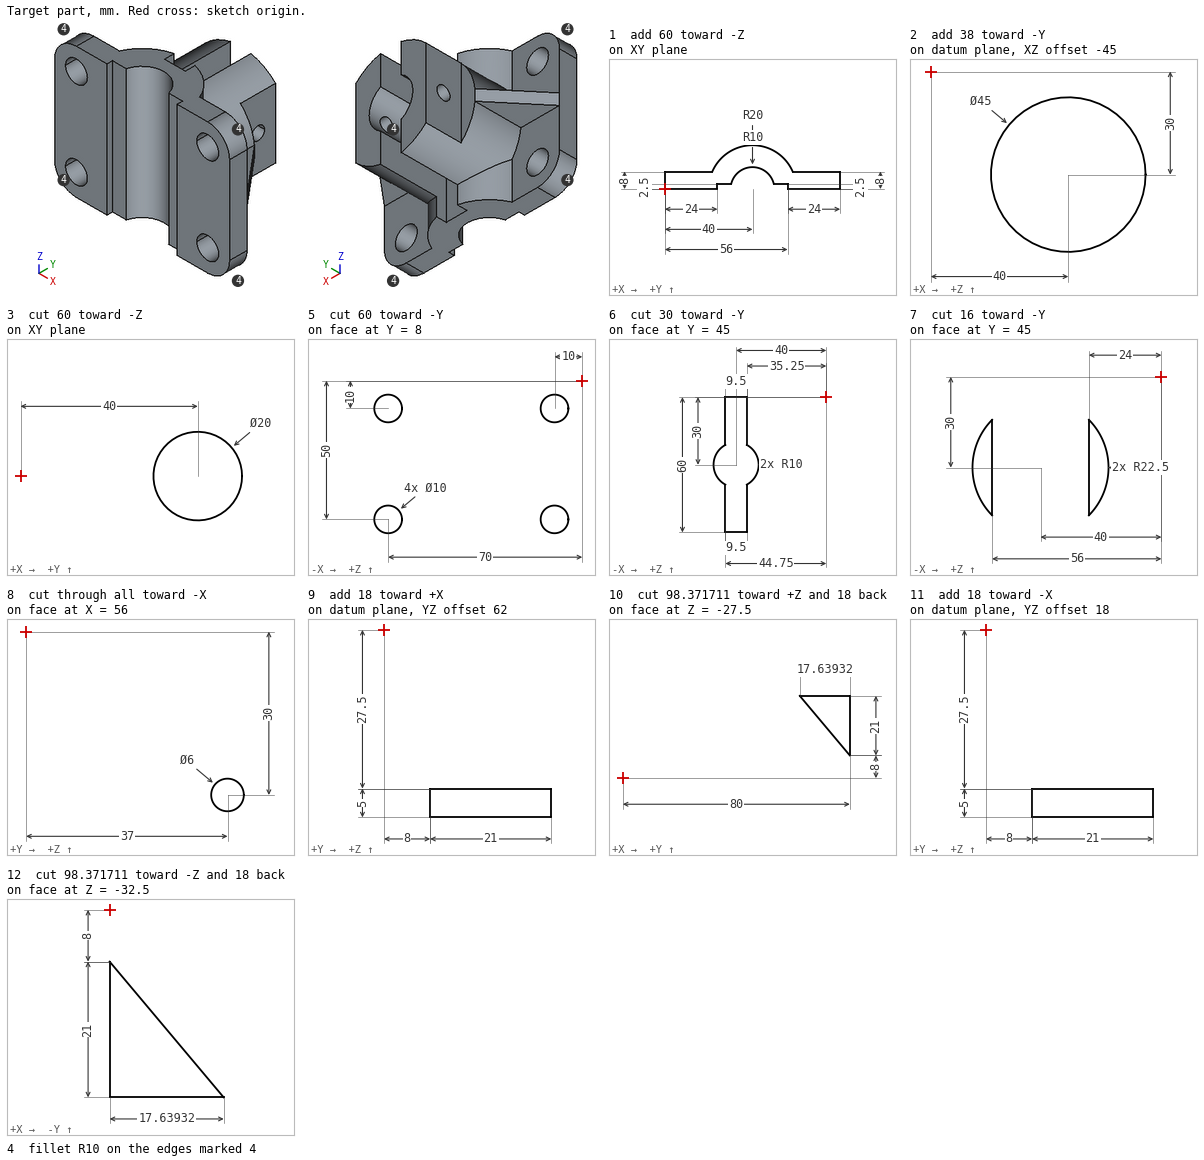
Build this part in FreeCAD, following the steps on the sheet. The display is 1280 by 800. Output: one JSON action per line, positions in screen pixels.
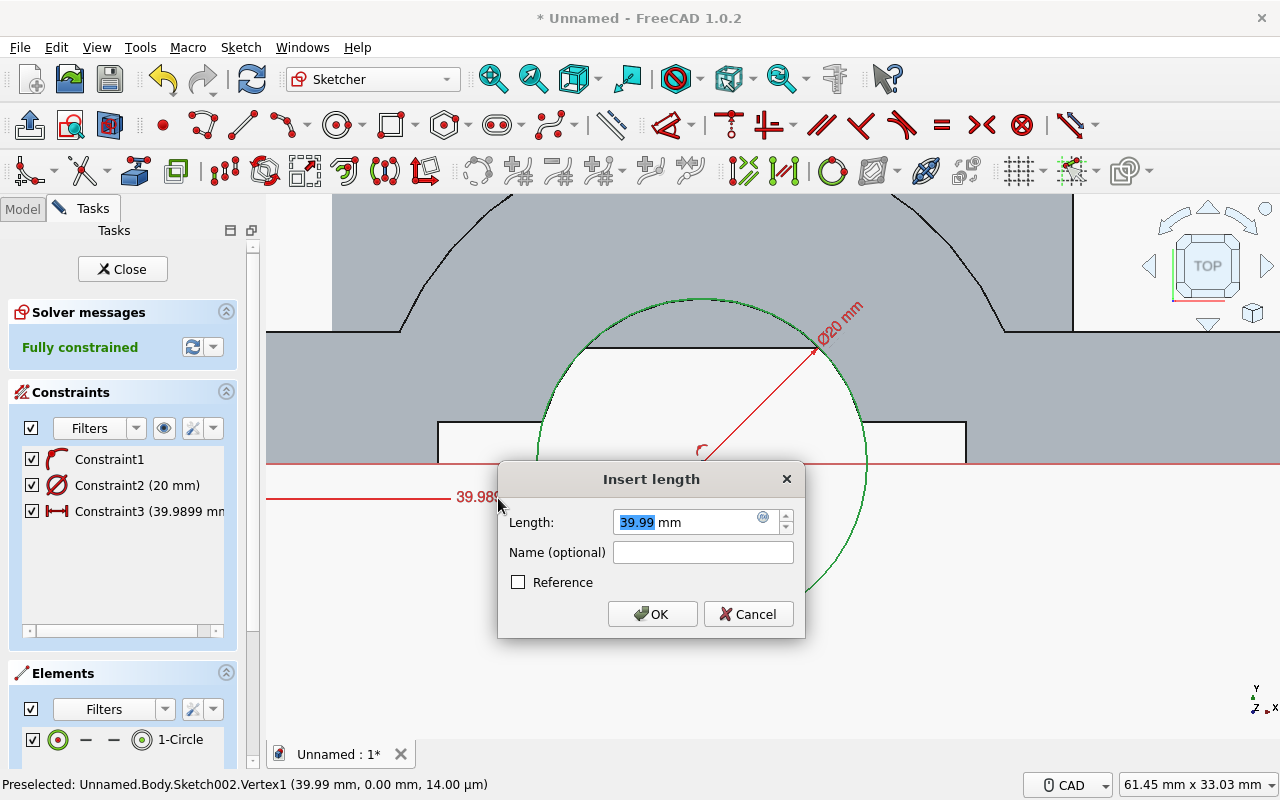
{"action": "type", "text": "40"}
{"action": "key", "text": "Return"}
{"action": "key", "text": "Escape"}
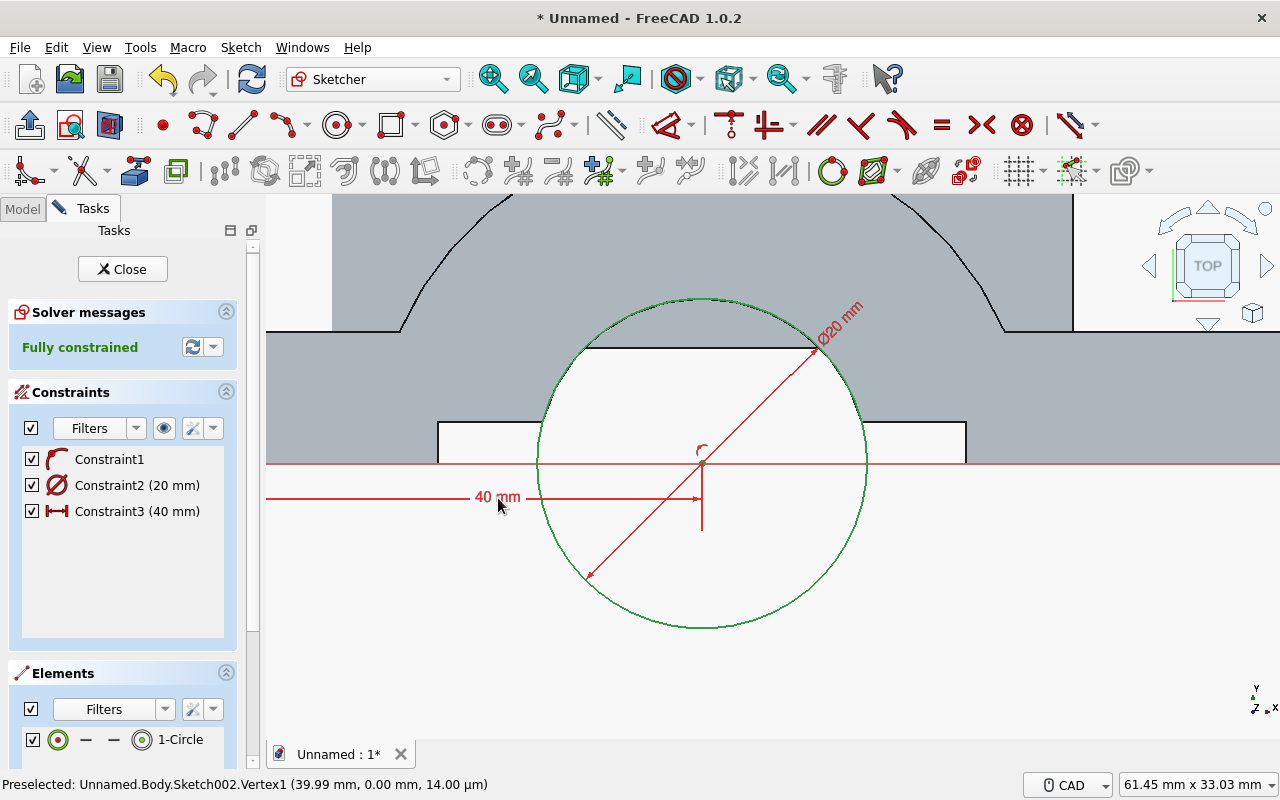
{"action": "left_click", "coordinate": [123, 269]}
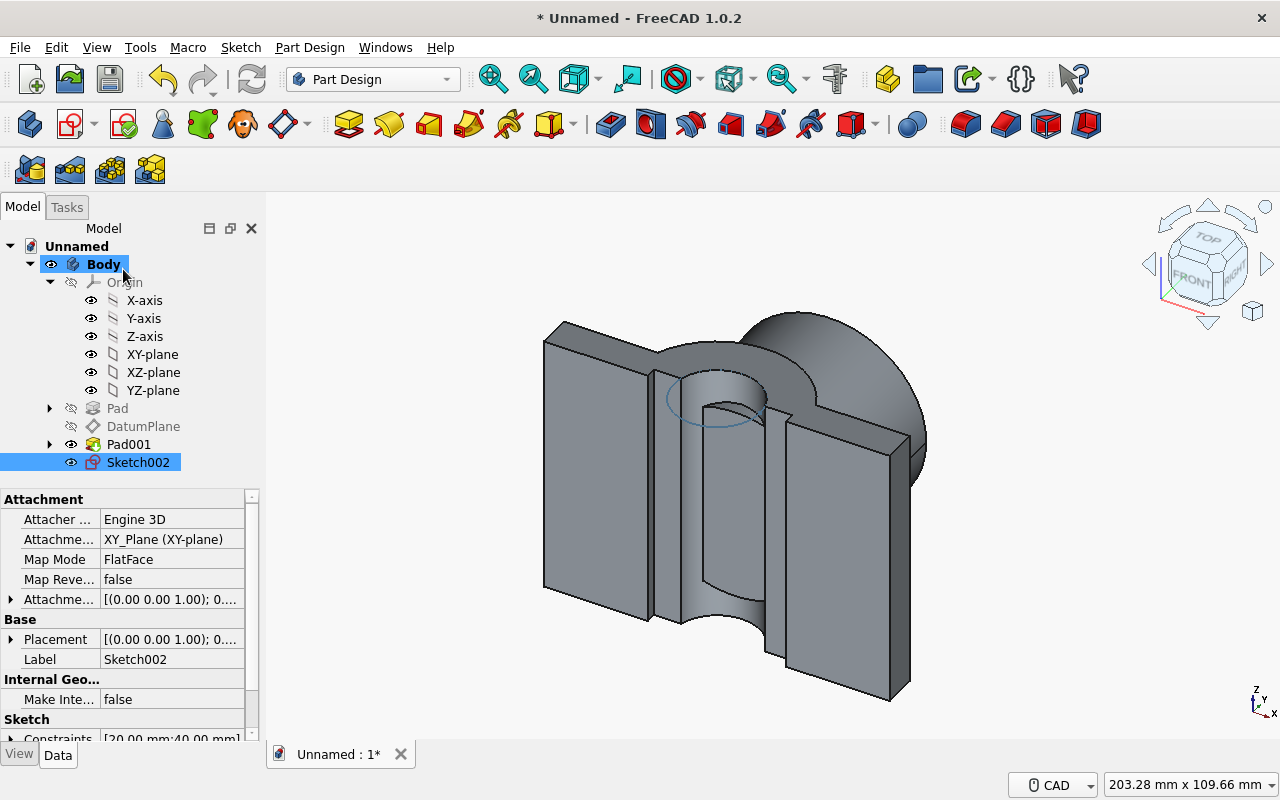
{"action": "left_click", "coordinate": [612, 124]}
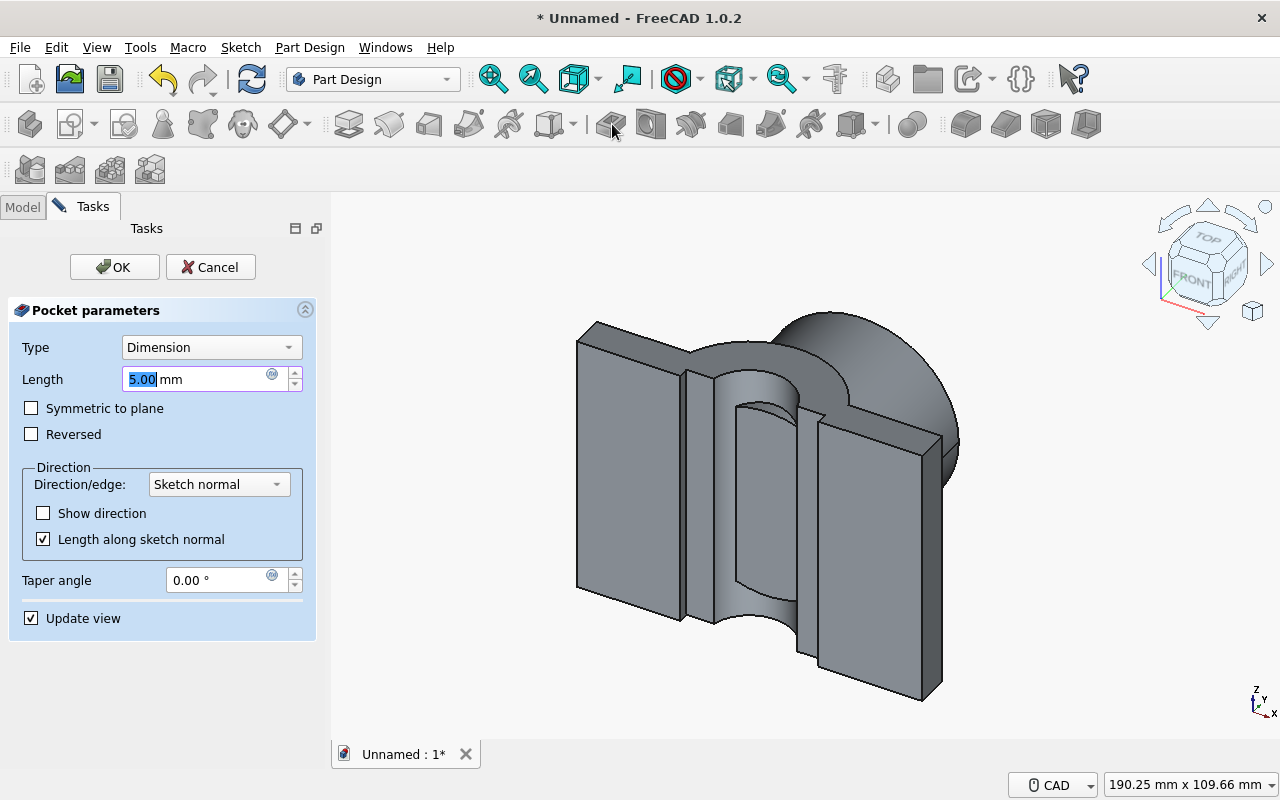
{"action": "type", "text": "60"}
{"action": "key", "text": "Tab"}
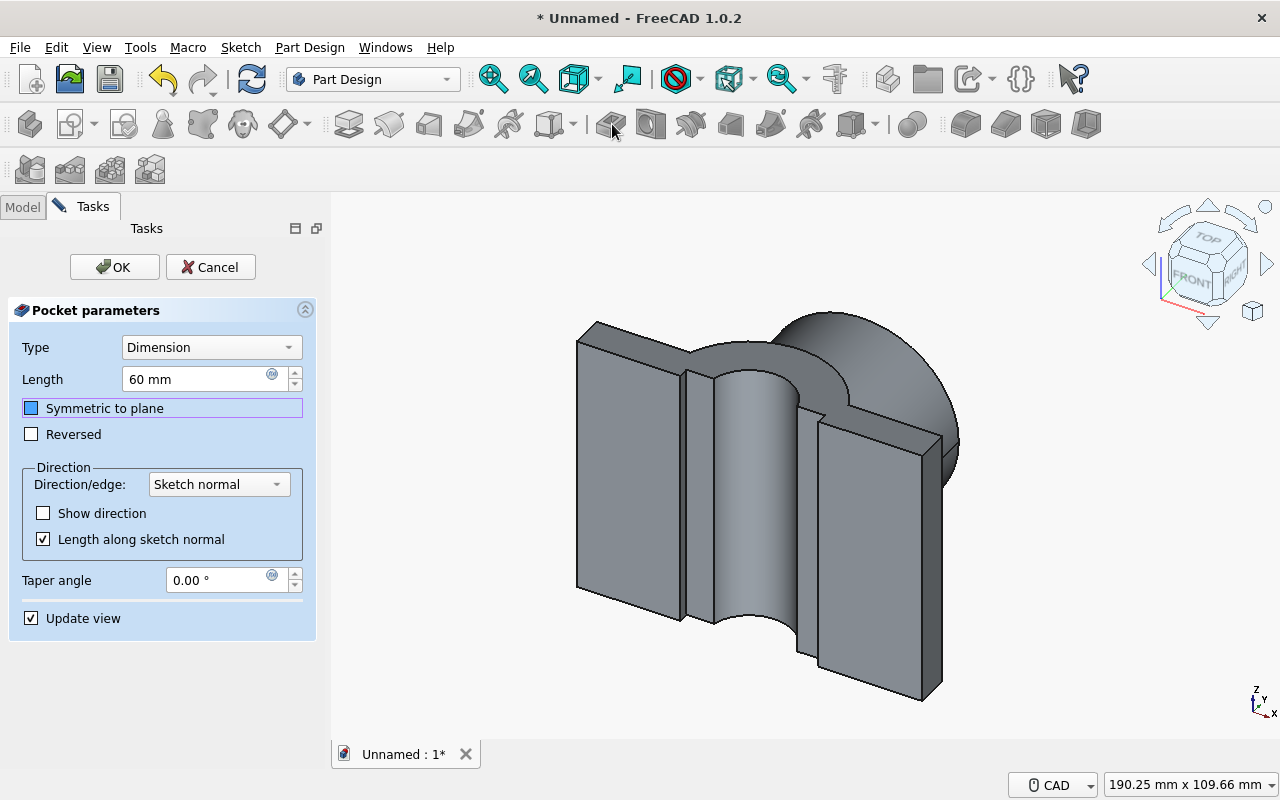
{"action": "left_click", "coordinate": [115, 267]}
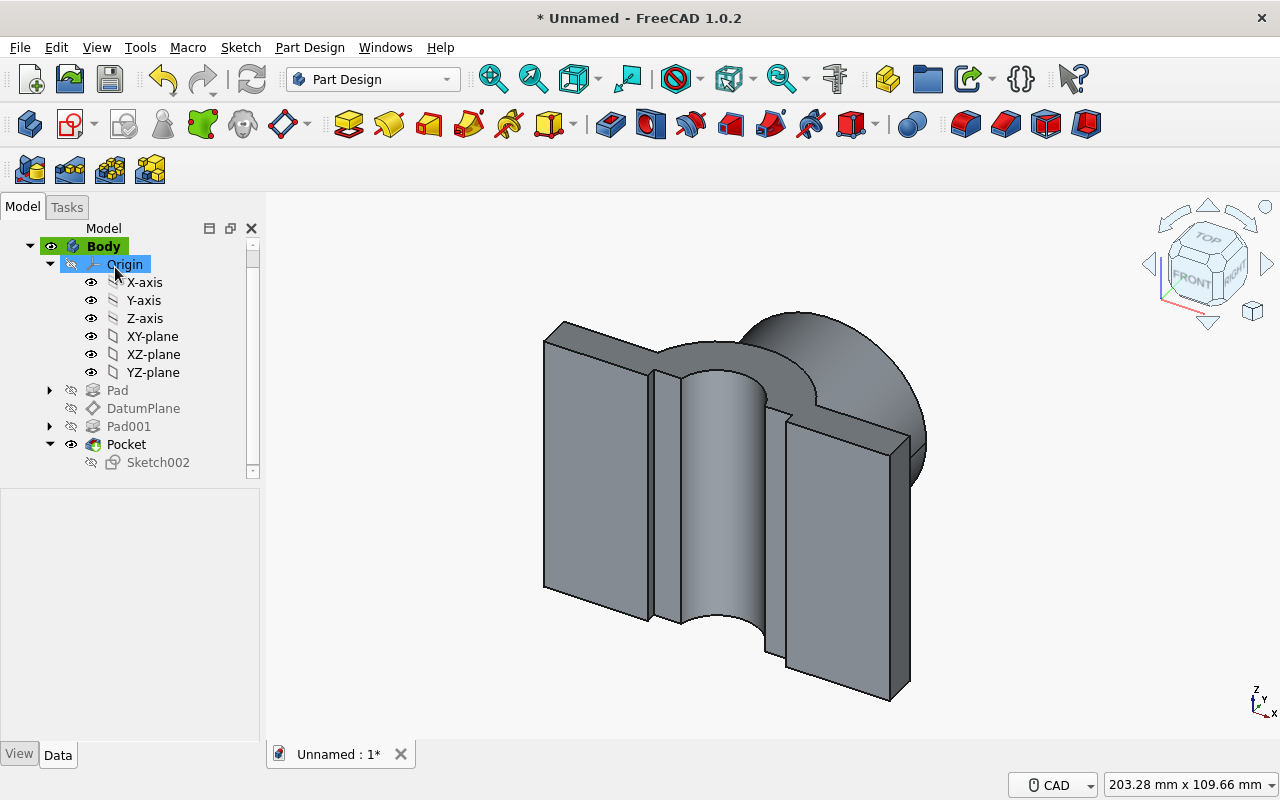
{"action": "left_click", "coordinate": [900, 445]}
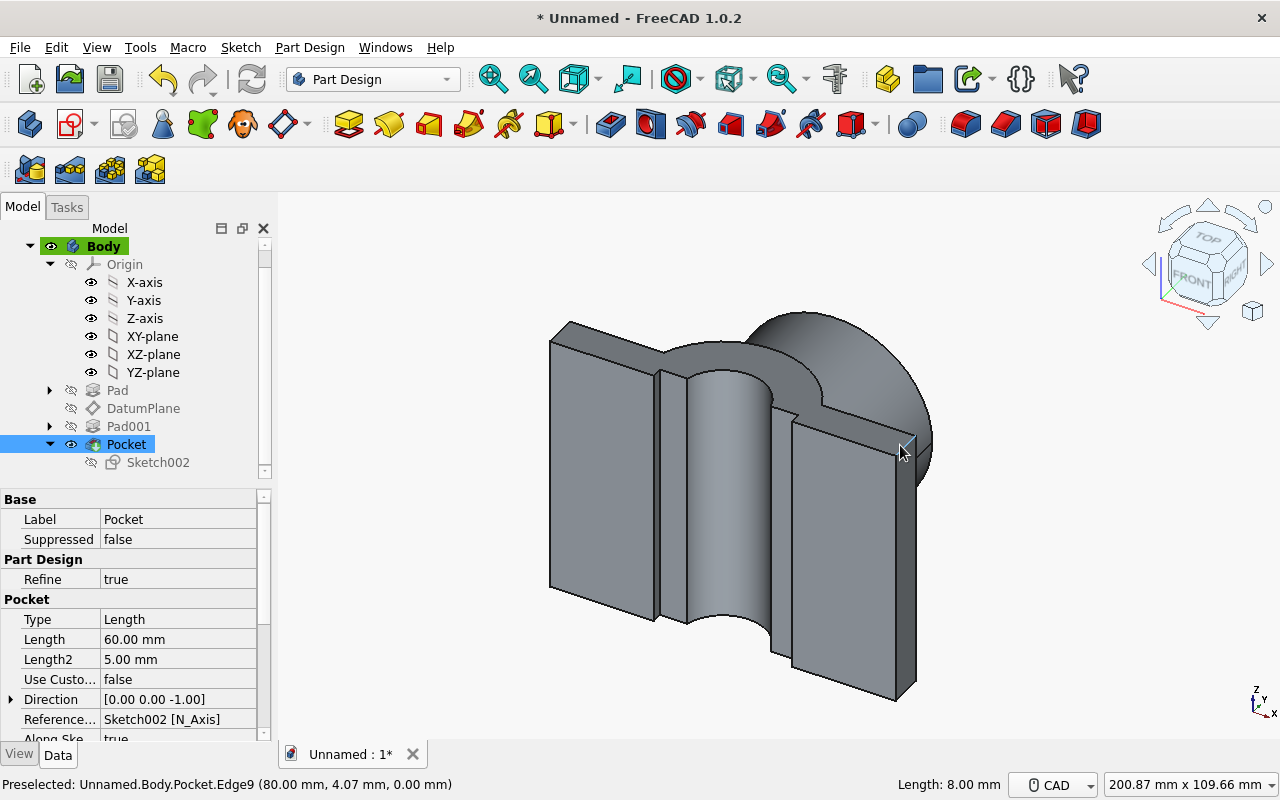
{"action": "key", "text": "0"}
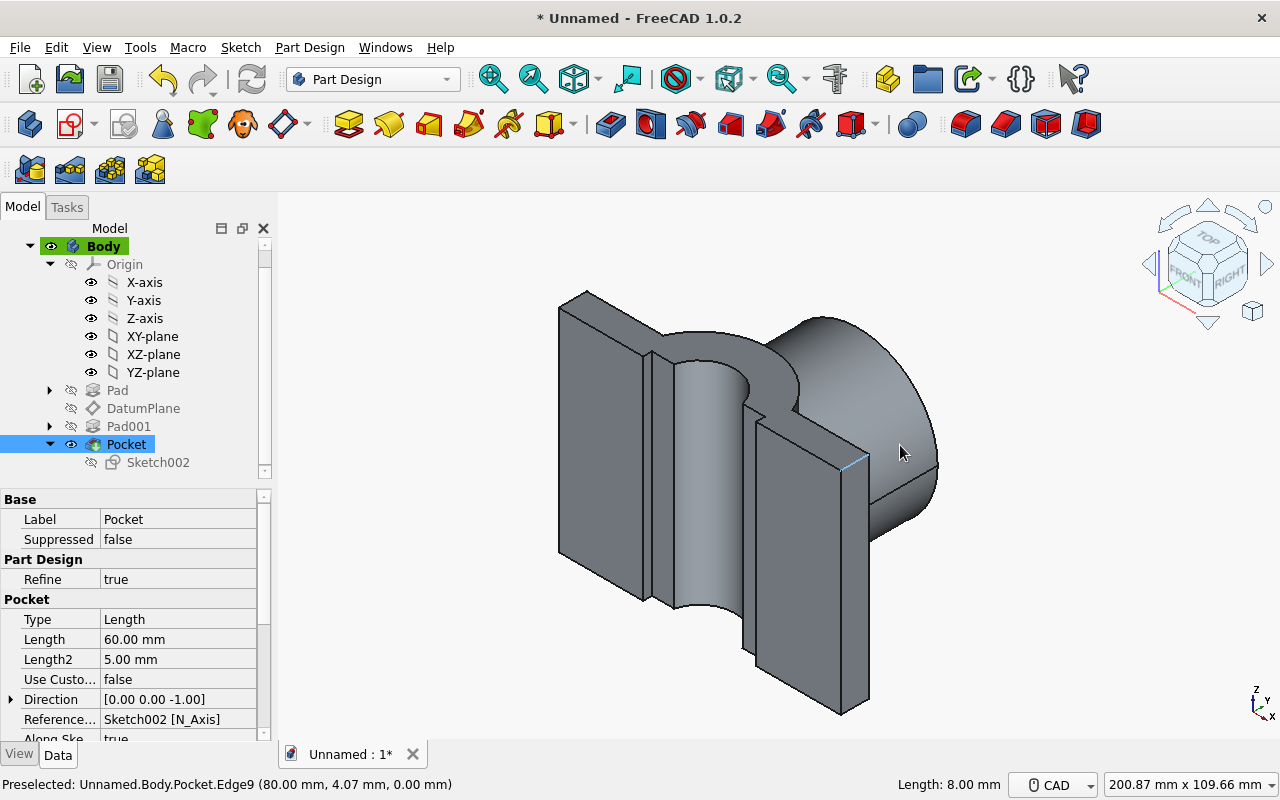
{"action": "key", "text": "2"}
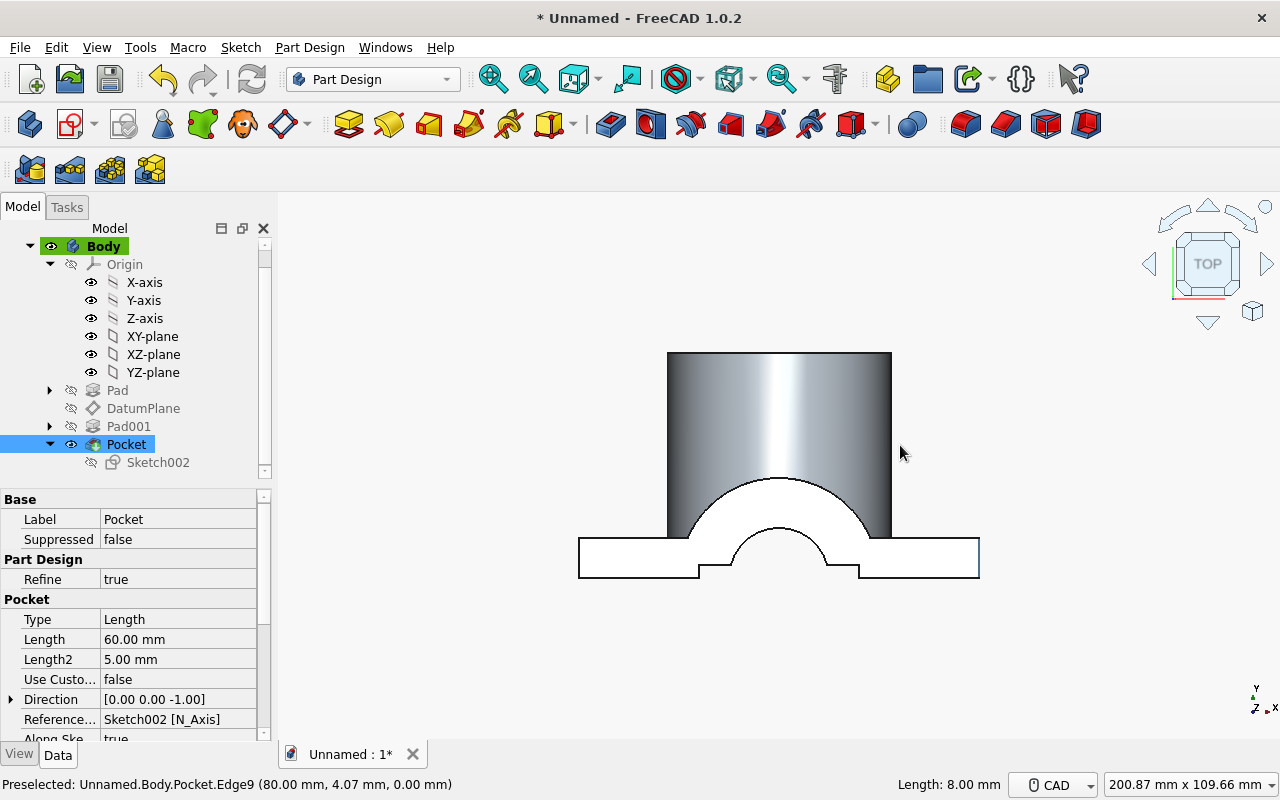
{"action": "left_click", "coordinate": [494, 80]}